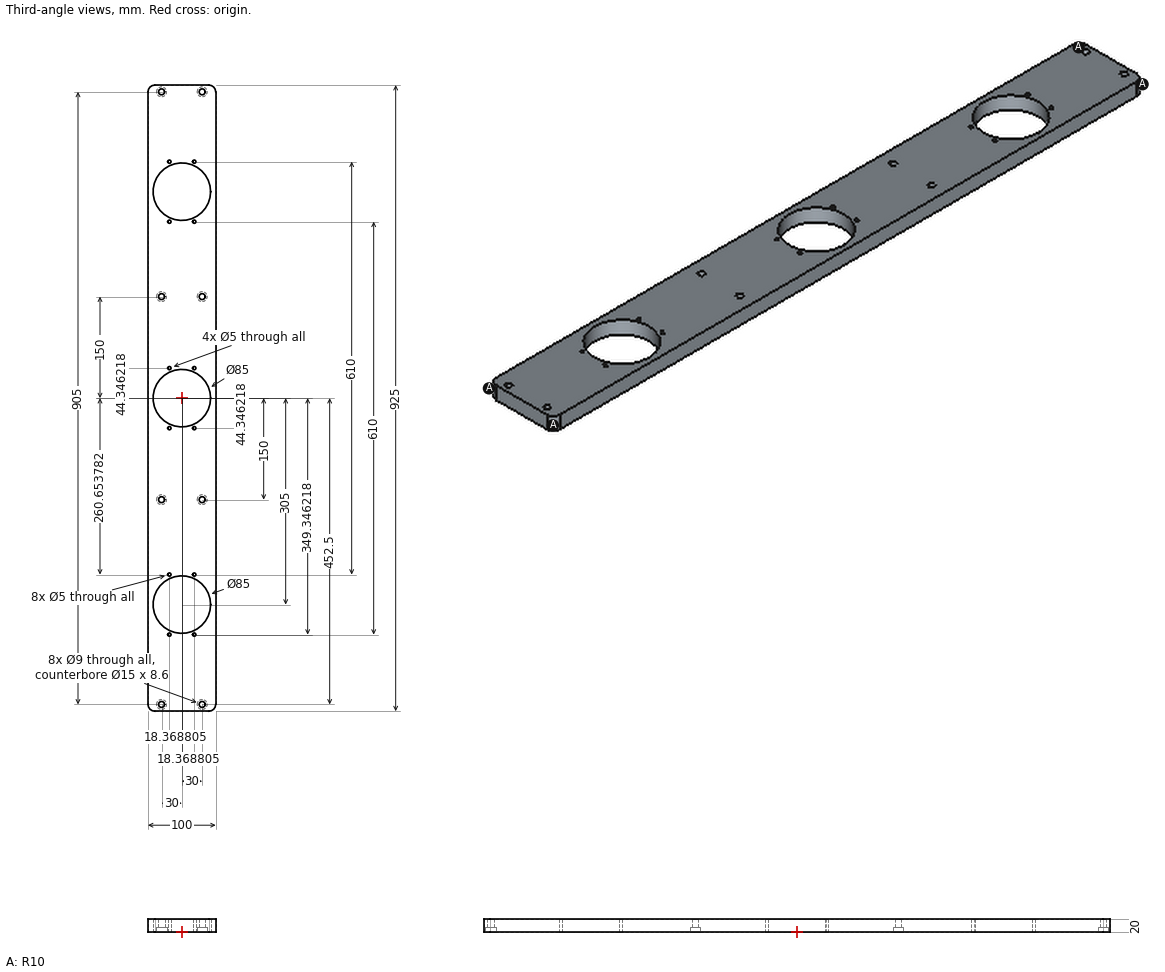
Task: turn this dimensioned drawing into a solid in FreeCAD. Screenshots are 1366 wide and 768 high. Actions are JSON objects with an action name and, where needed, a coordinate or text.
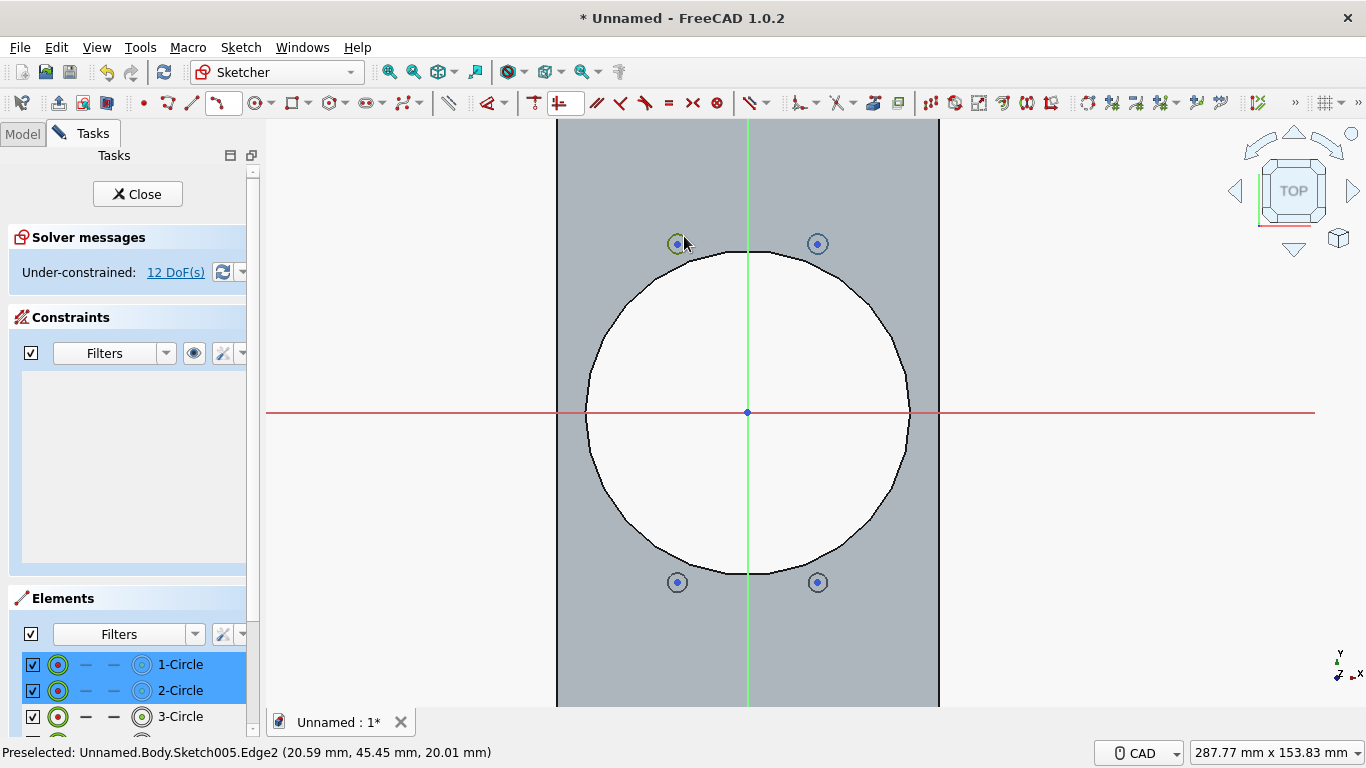
{"action": "scroll", "coordinate": [825, 576], "scroll_direction": "up", "scroll_amount": 2}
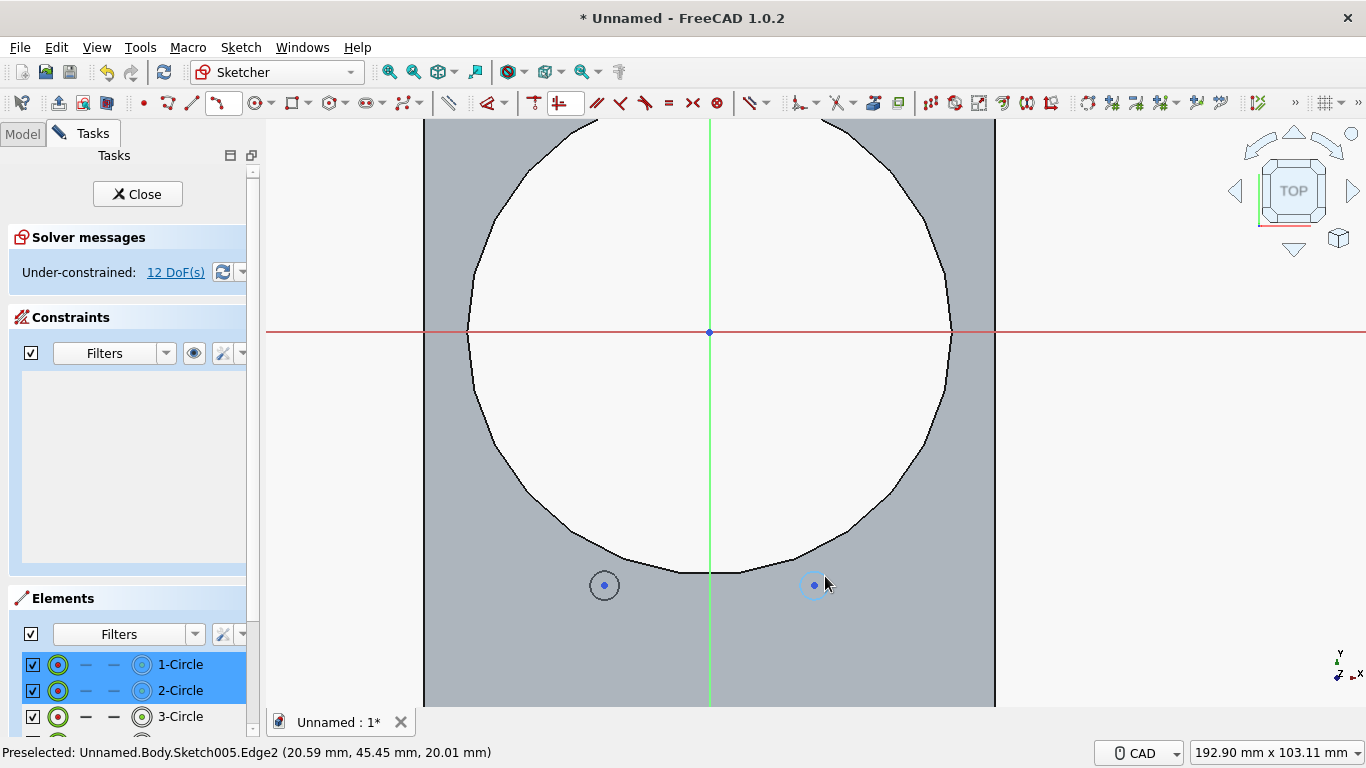
{"action": "left_click", "coordinate": [824, 576]}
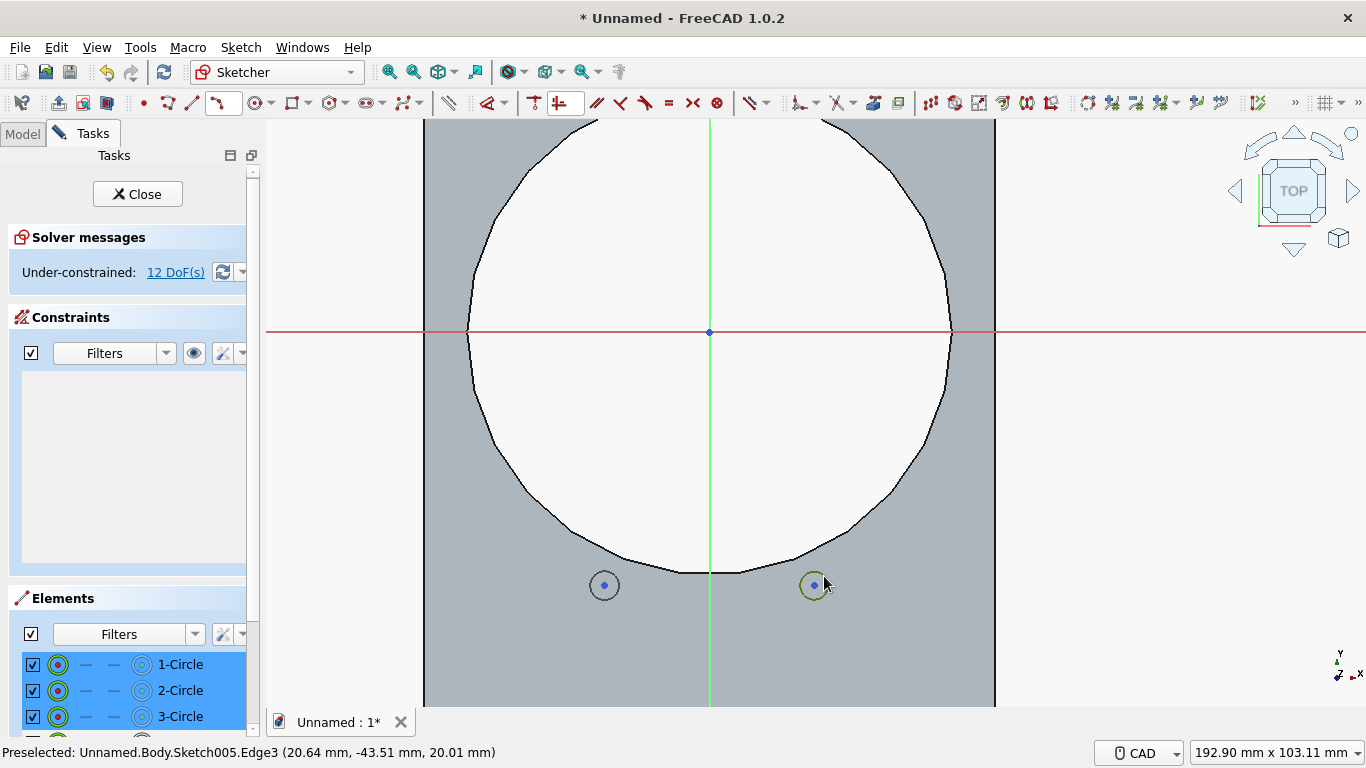
{"action": "left_click", "coordinate": [615, 575]}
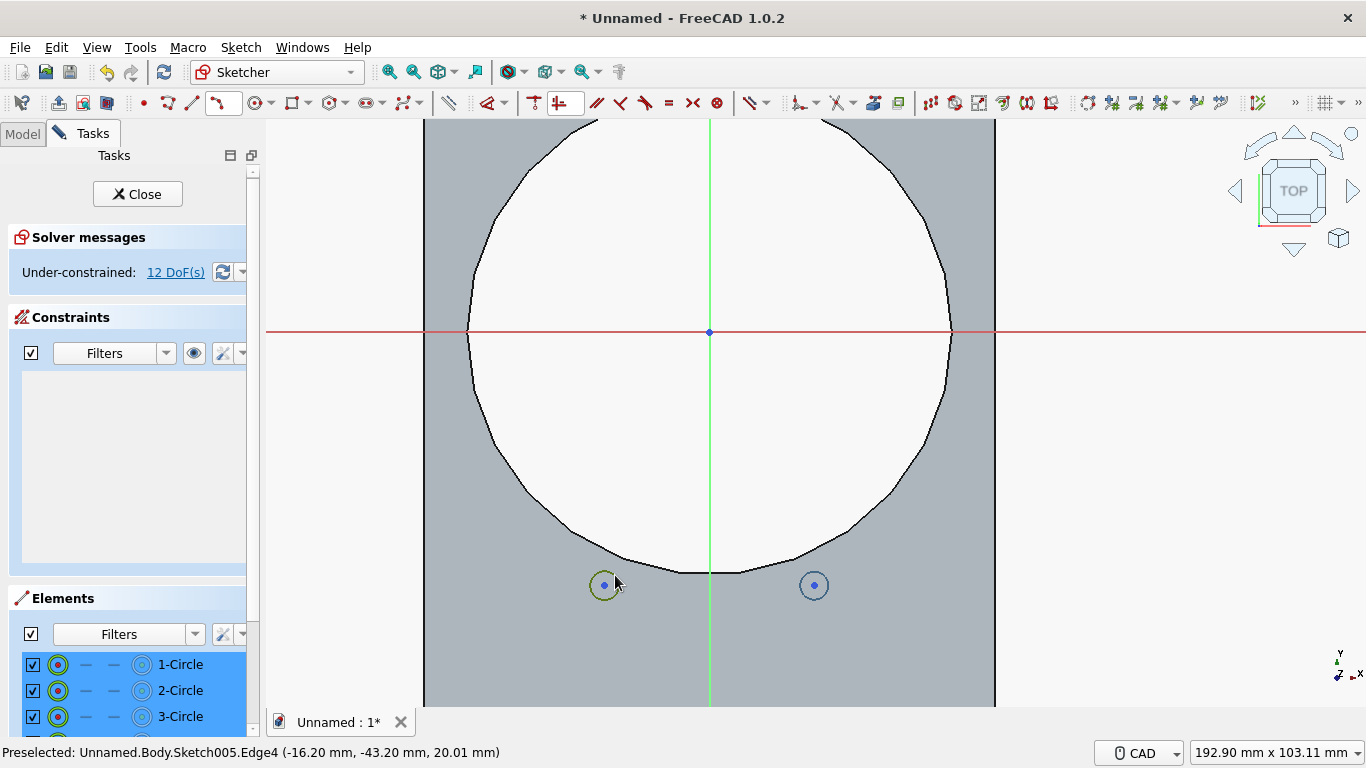
{"action": "key", "text": "e"}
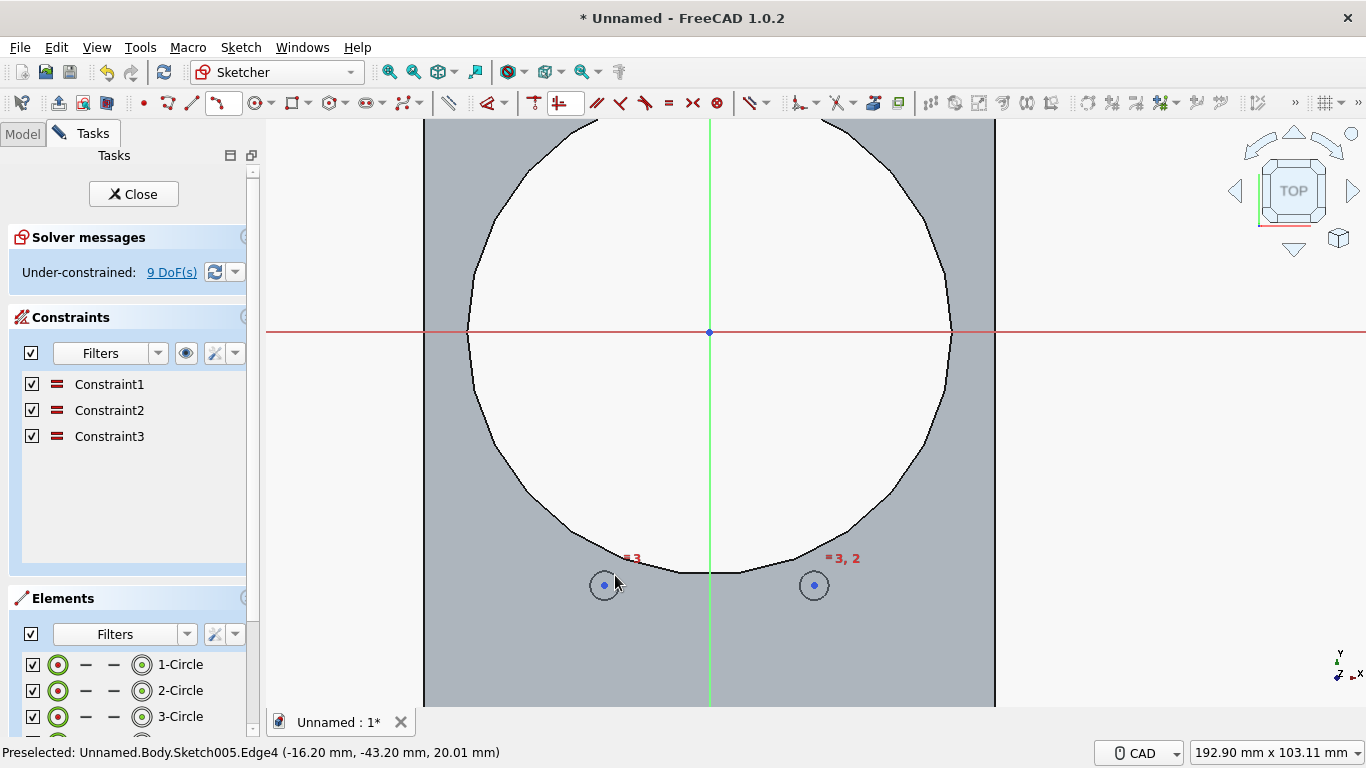
{"action": "left_click", "coordinate": [488, 104]}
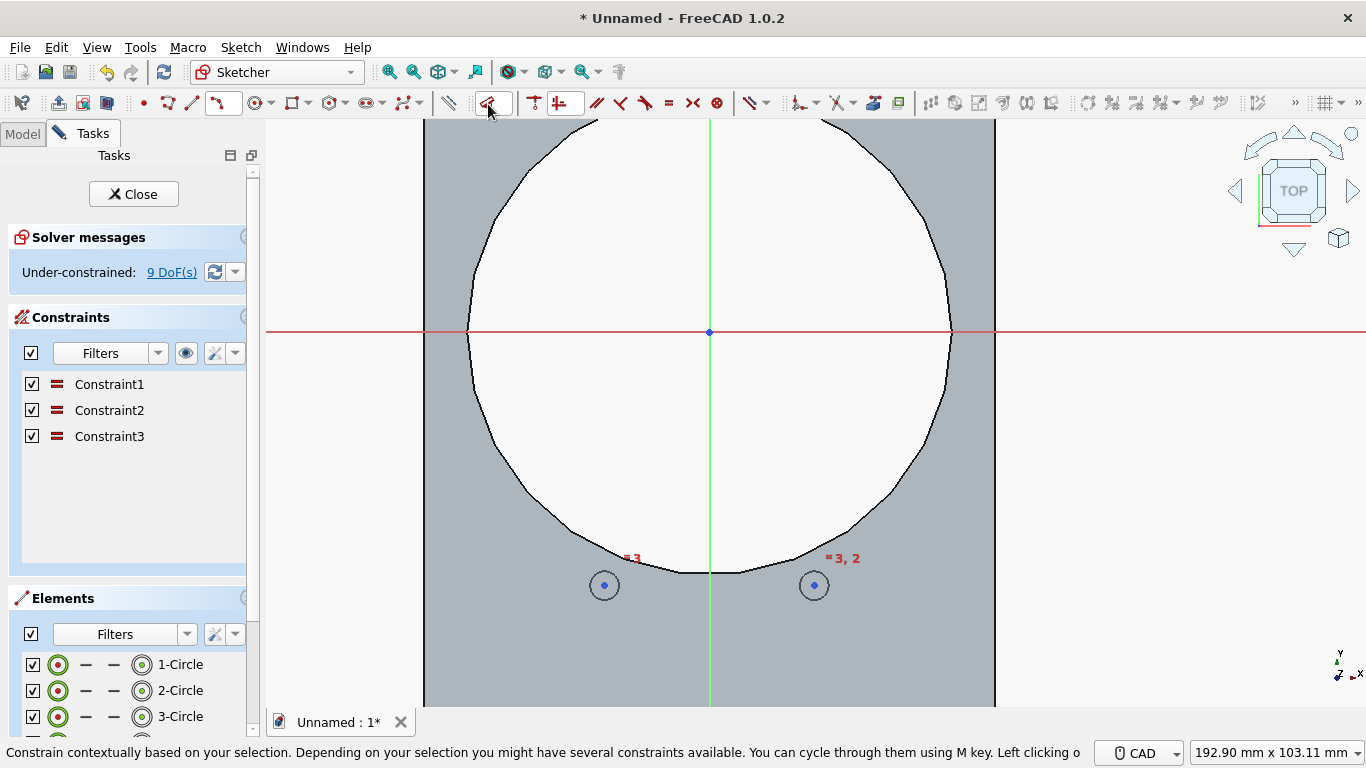
{"action": "scroll", "coordinate": [825, 577], "scroll_direction": "down", "scroll_amount": 2}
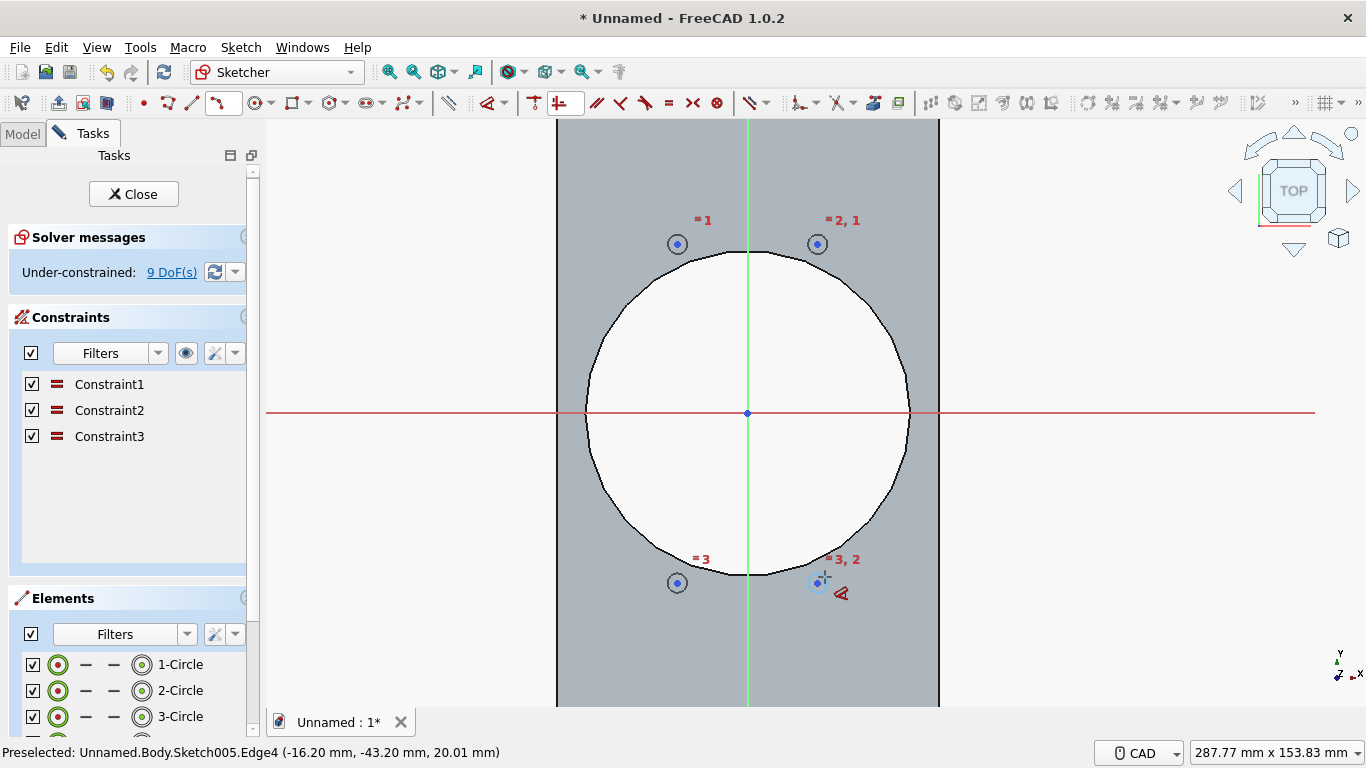
{"action": "scroll", "coordinate": [684, 238], "scroll_direction": "up", "scroll_amount": 4}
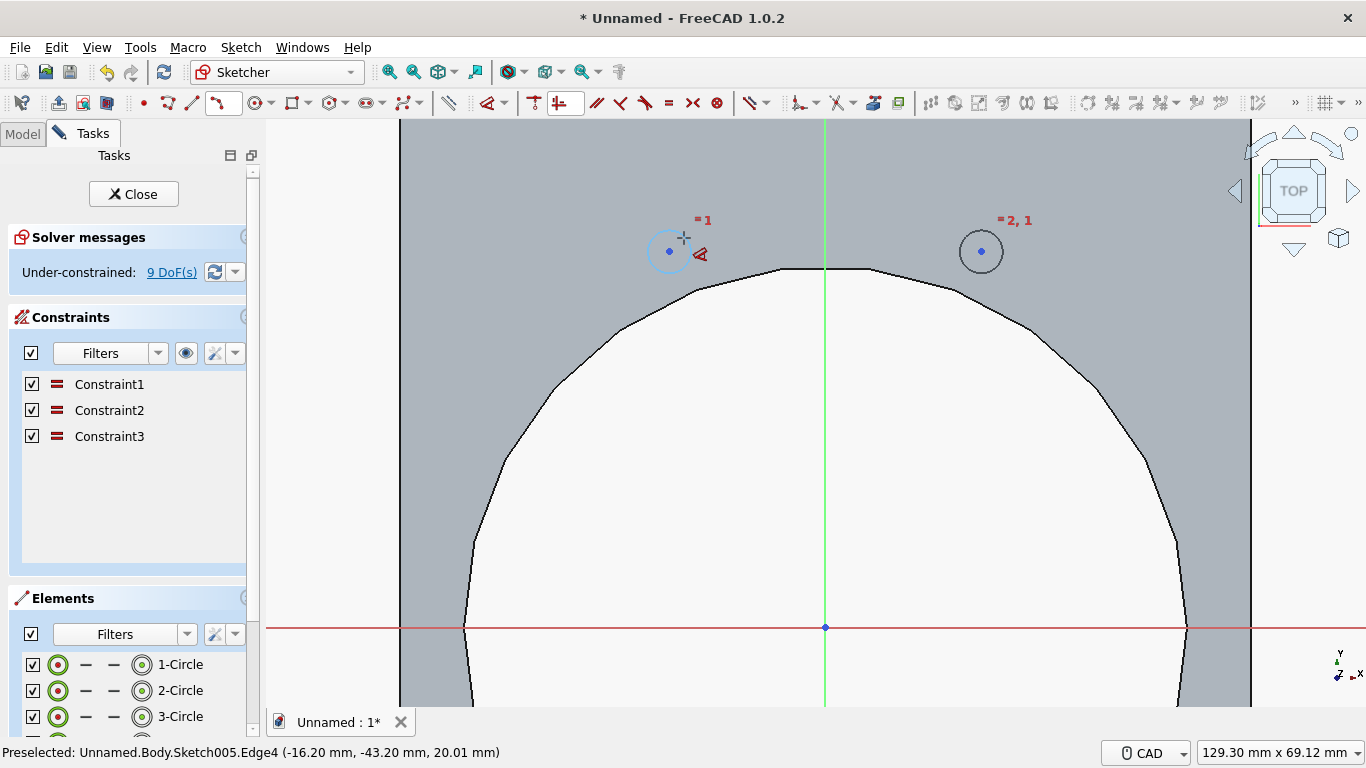
{"action": "left_click", "coordinate": [685, 237]}
{"action": "left_click", "coordinate": [708, 215]}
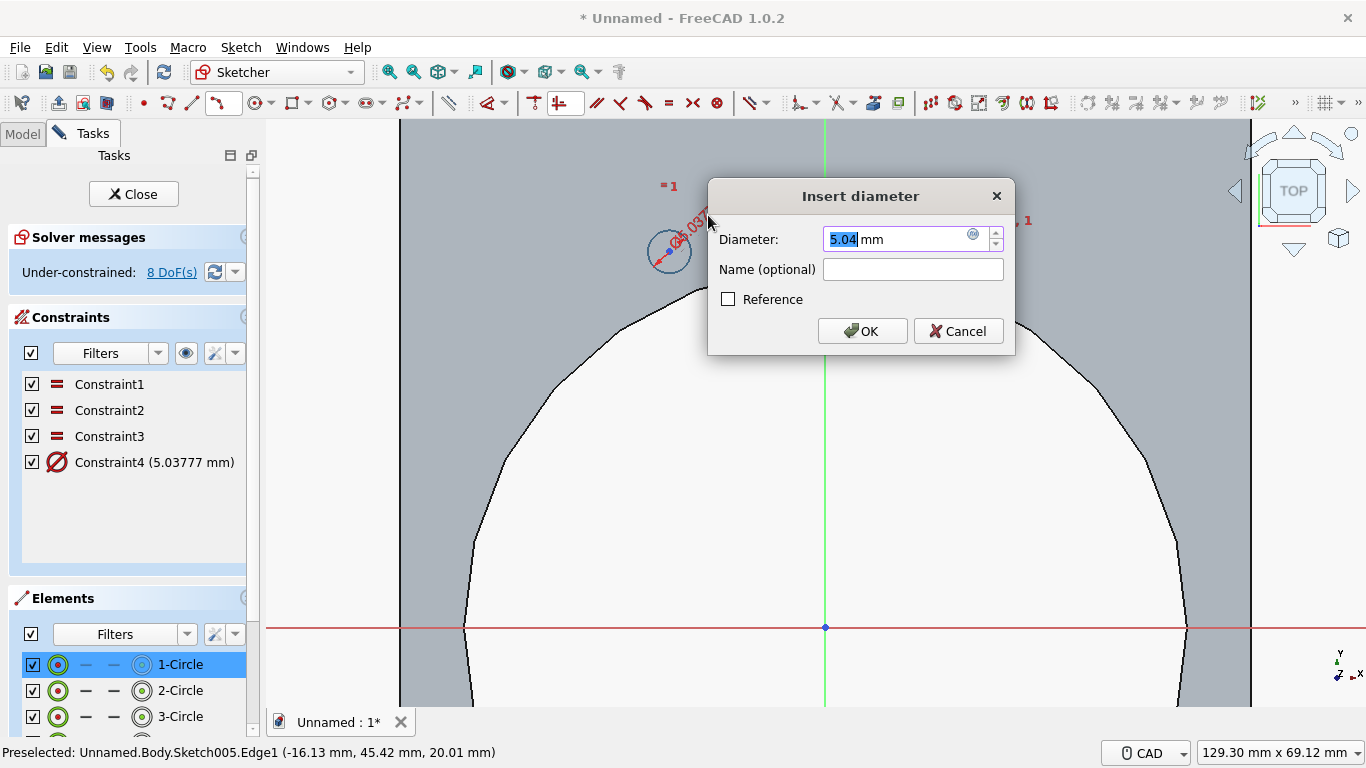
{"action": "type", "text": "5"}
{"action": "key", "text": "Return"}